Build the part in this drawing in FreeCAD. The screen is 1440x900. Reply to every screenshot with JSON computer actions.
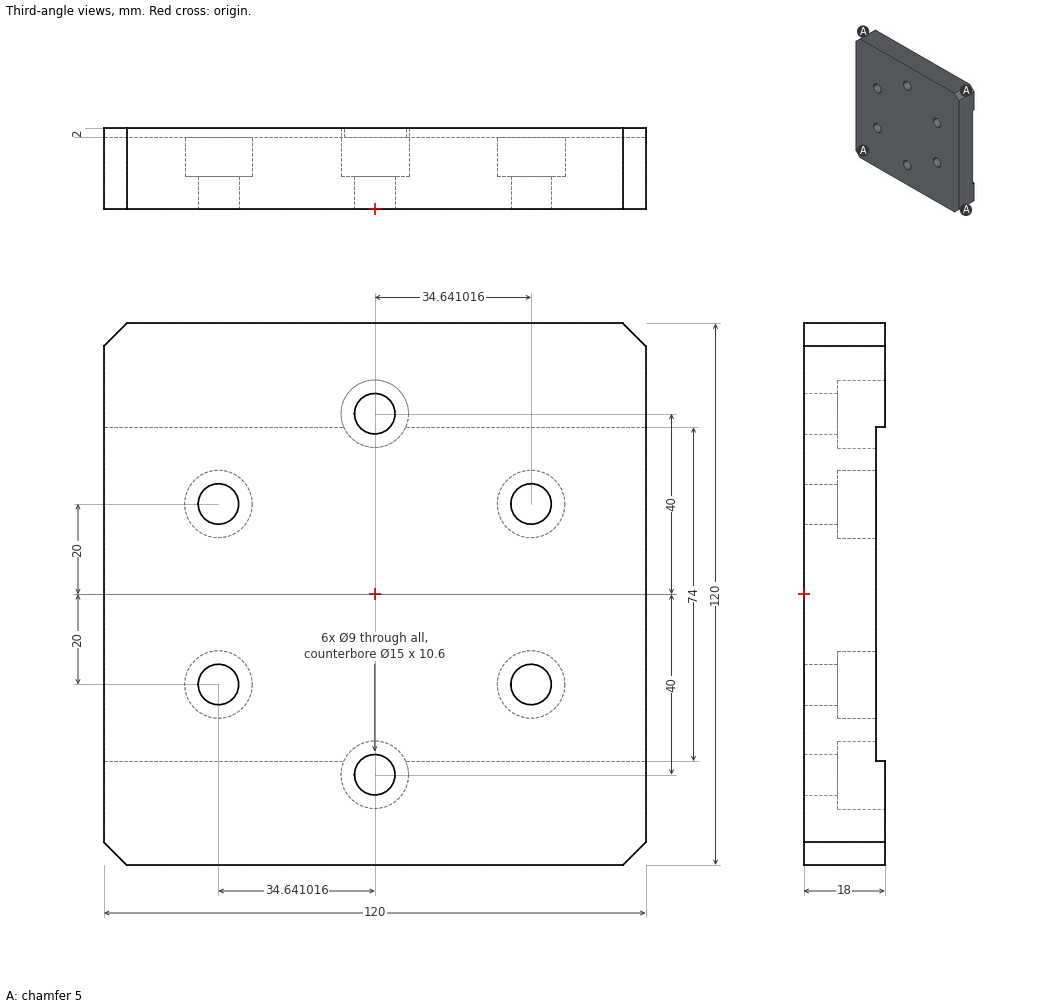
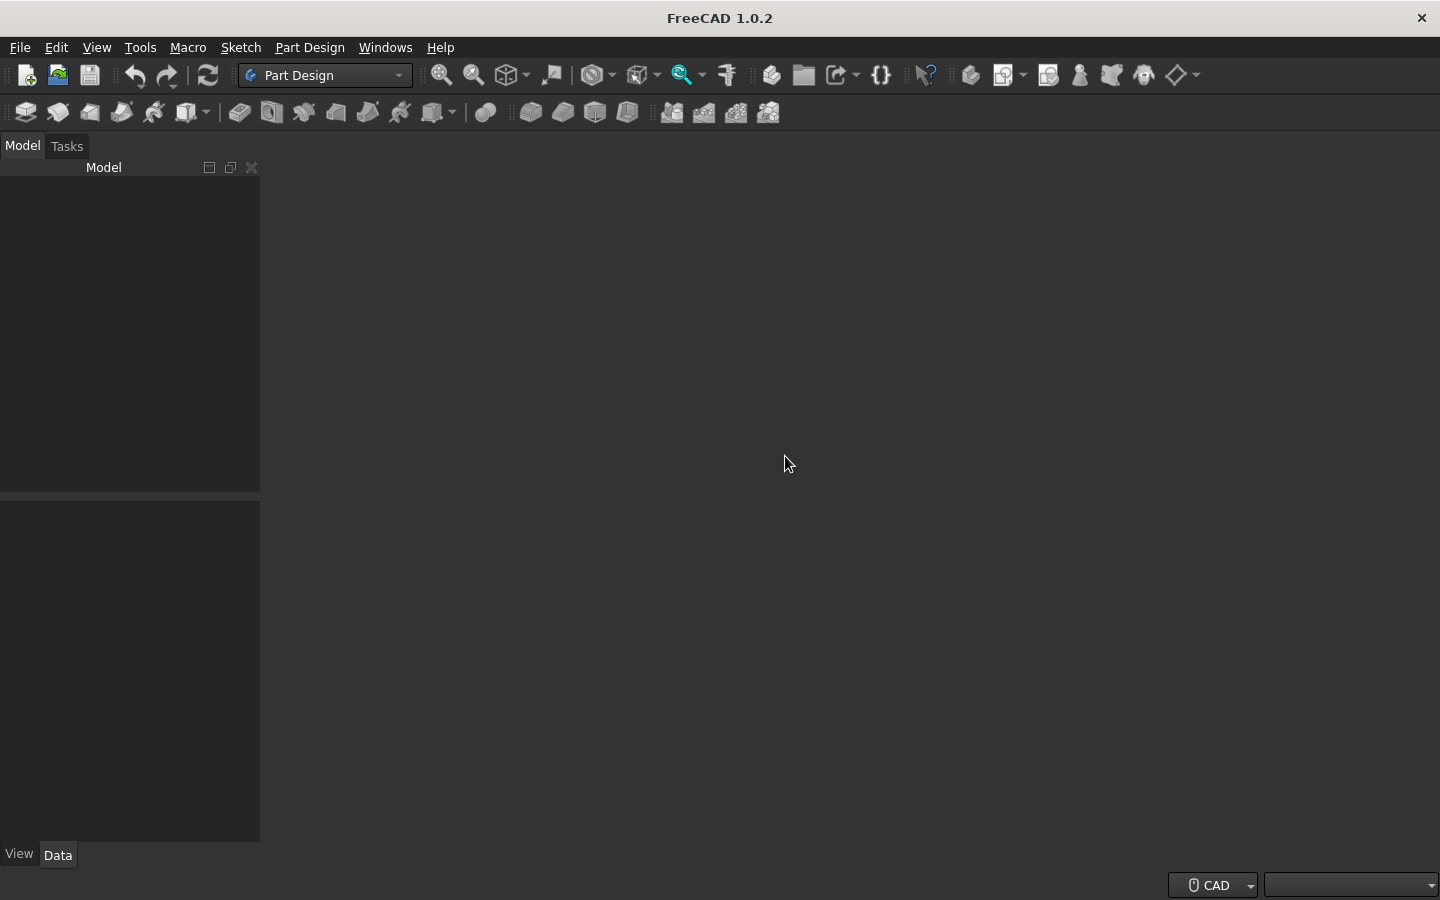
{"action": "left_click", "coordinate": [26, 76]}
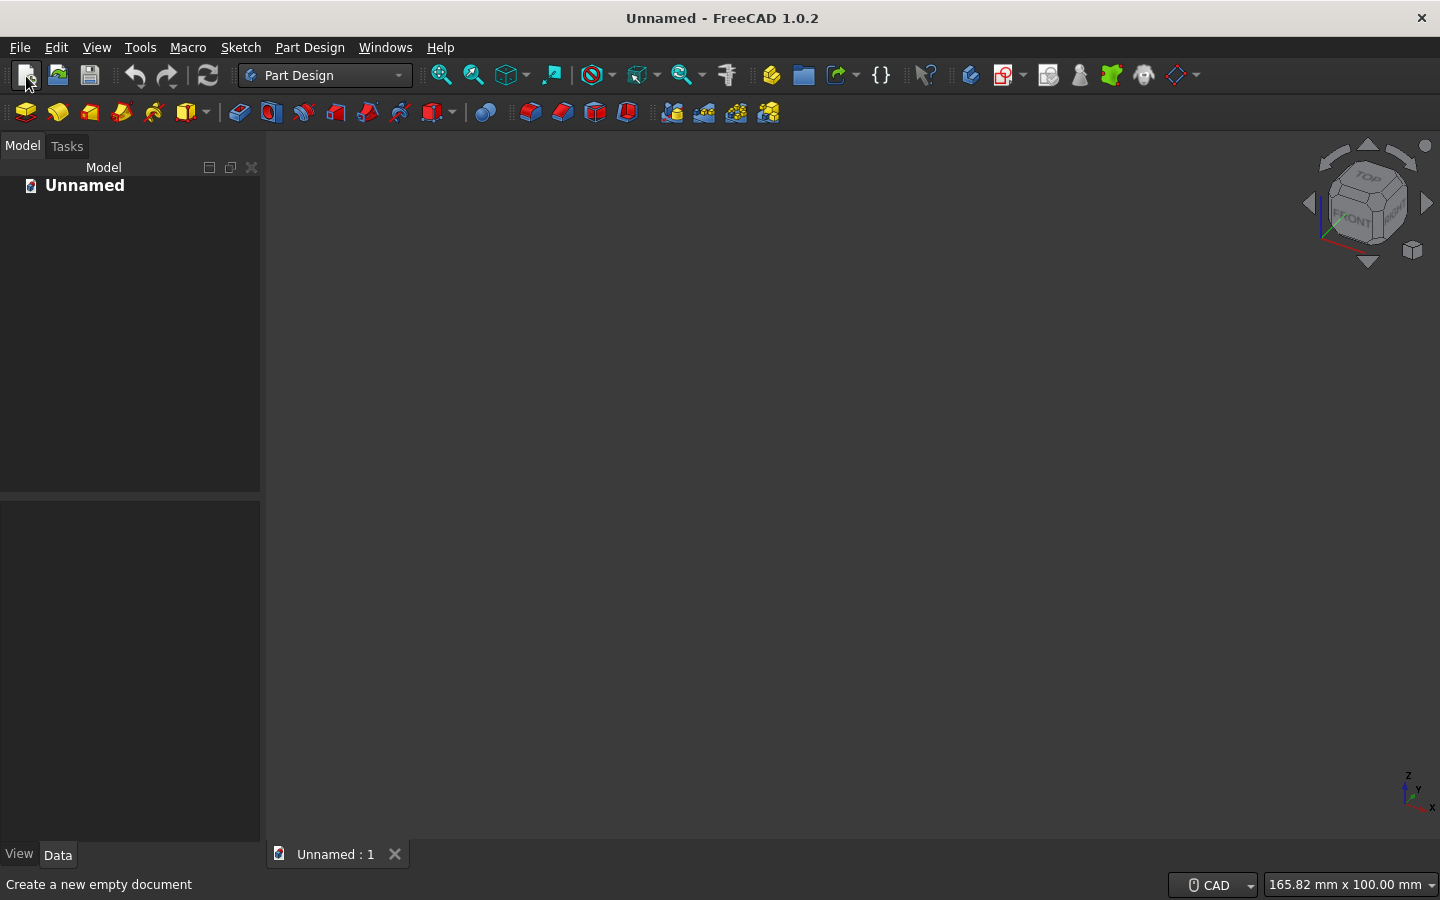
{"action": "left_click", "coordinate": [1004, 76]}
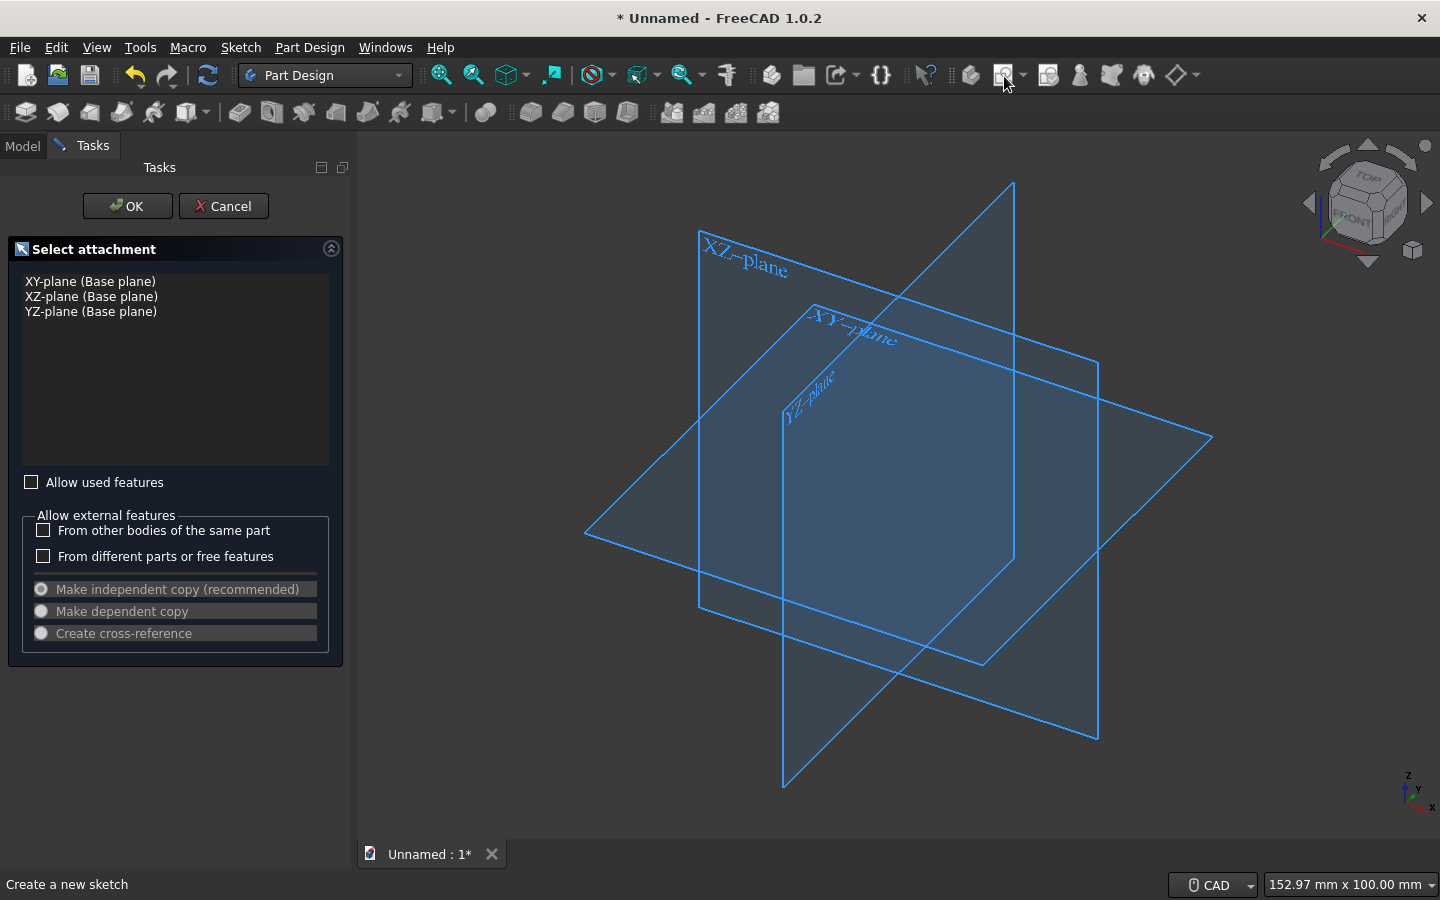
{"action": "left_click", "coordinate": [82, 296]}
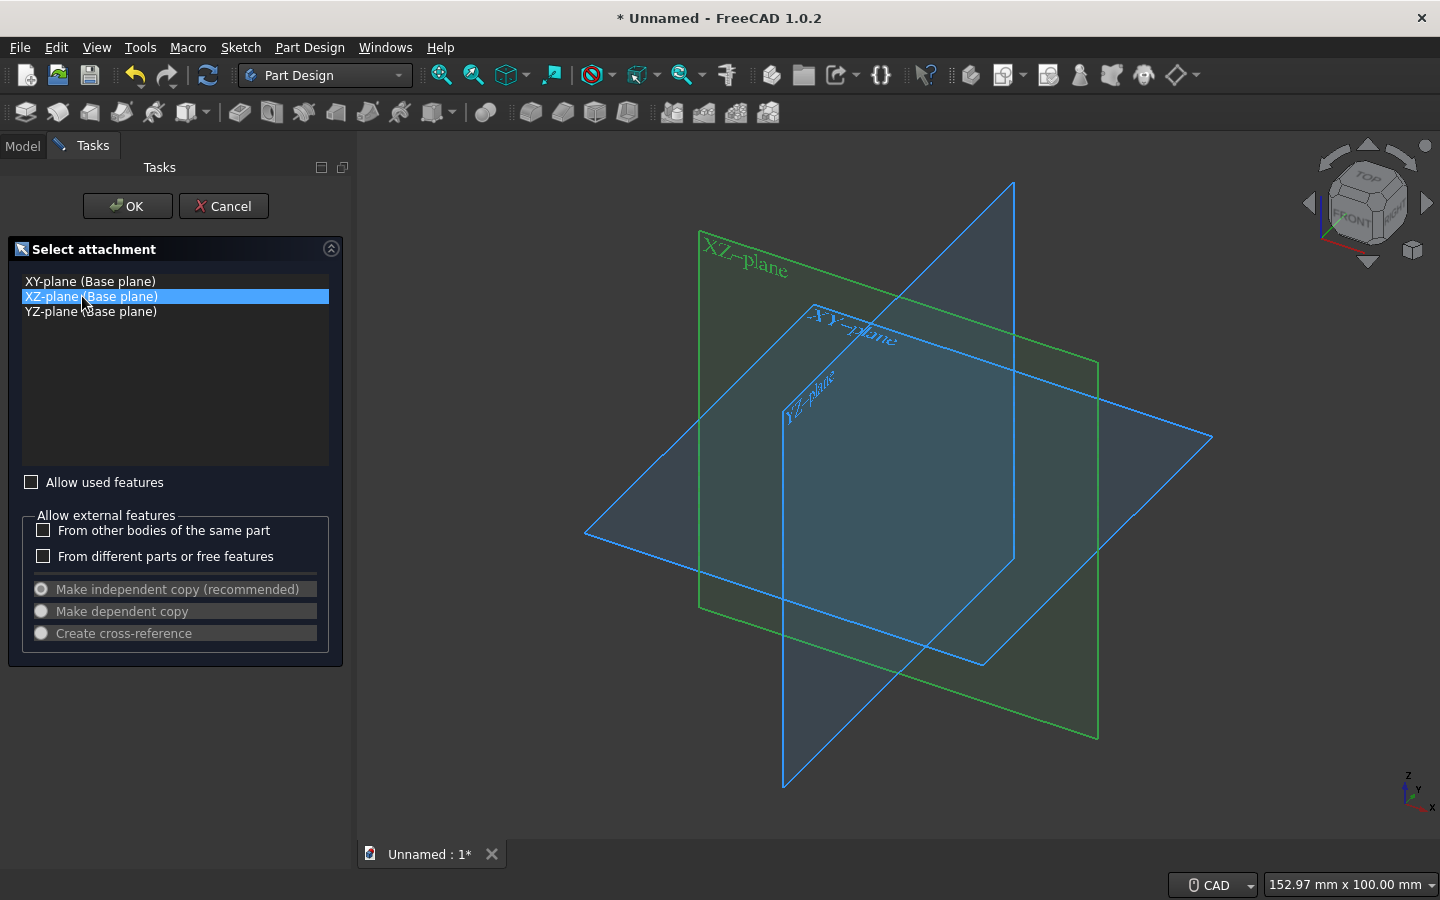
{"action": "left_click", "coordinate": [128, 206]}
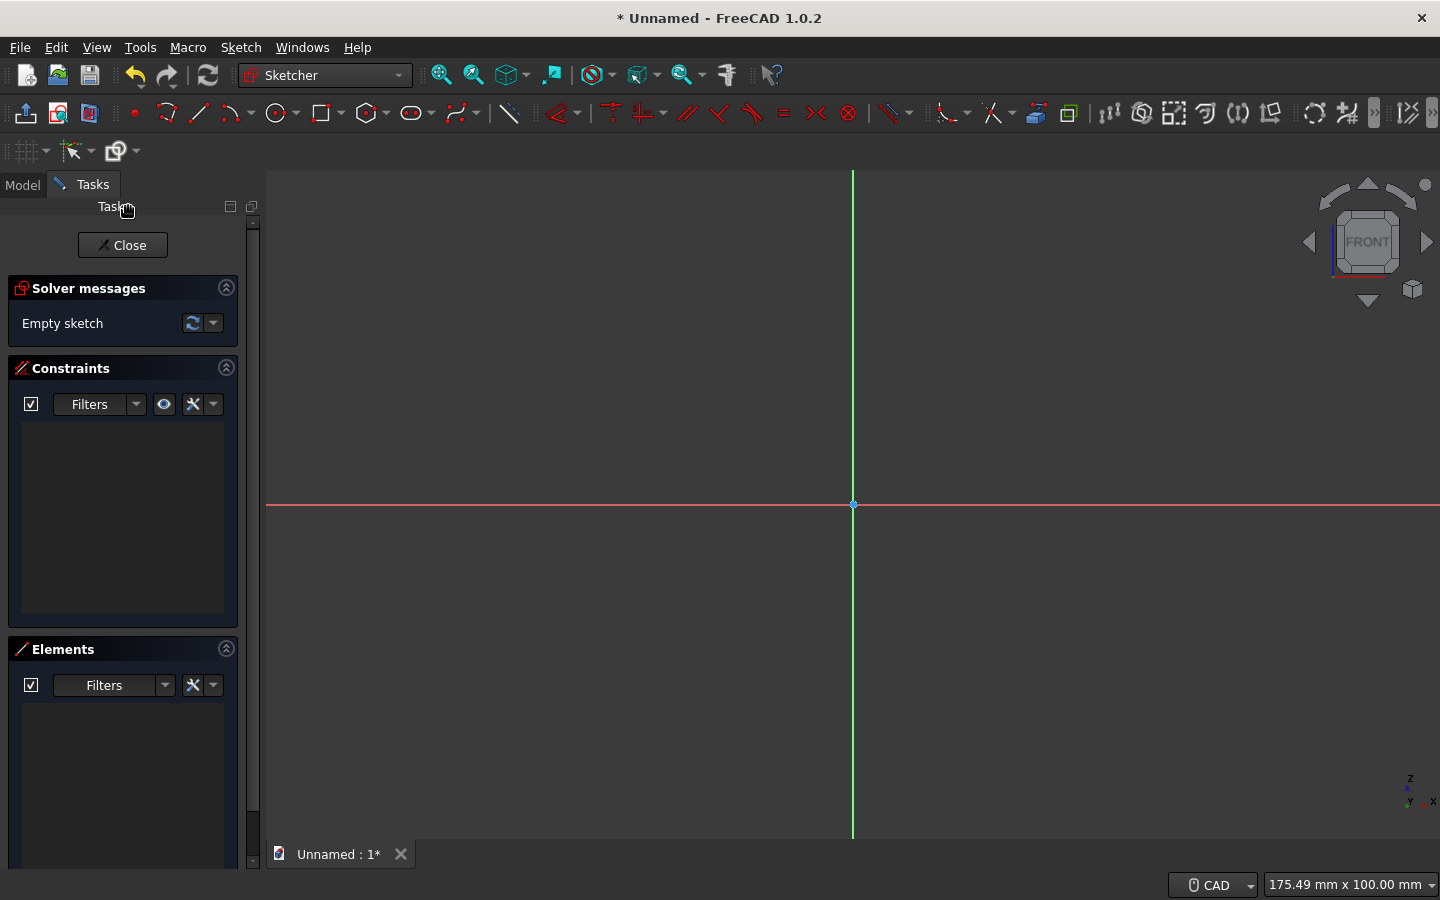
{"action": "scroll", "coordinate": [701, 504], "scroll_direction": "down", "scroll_amount": 3}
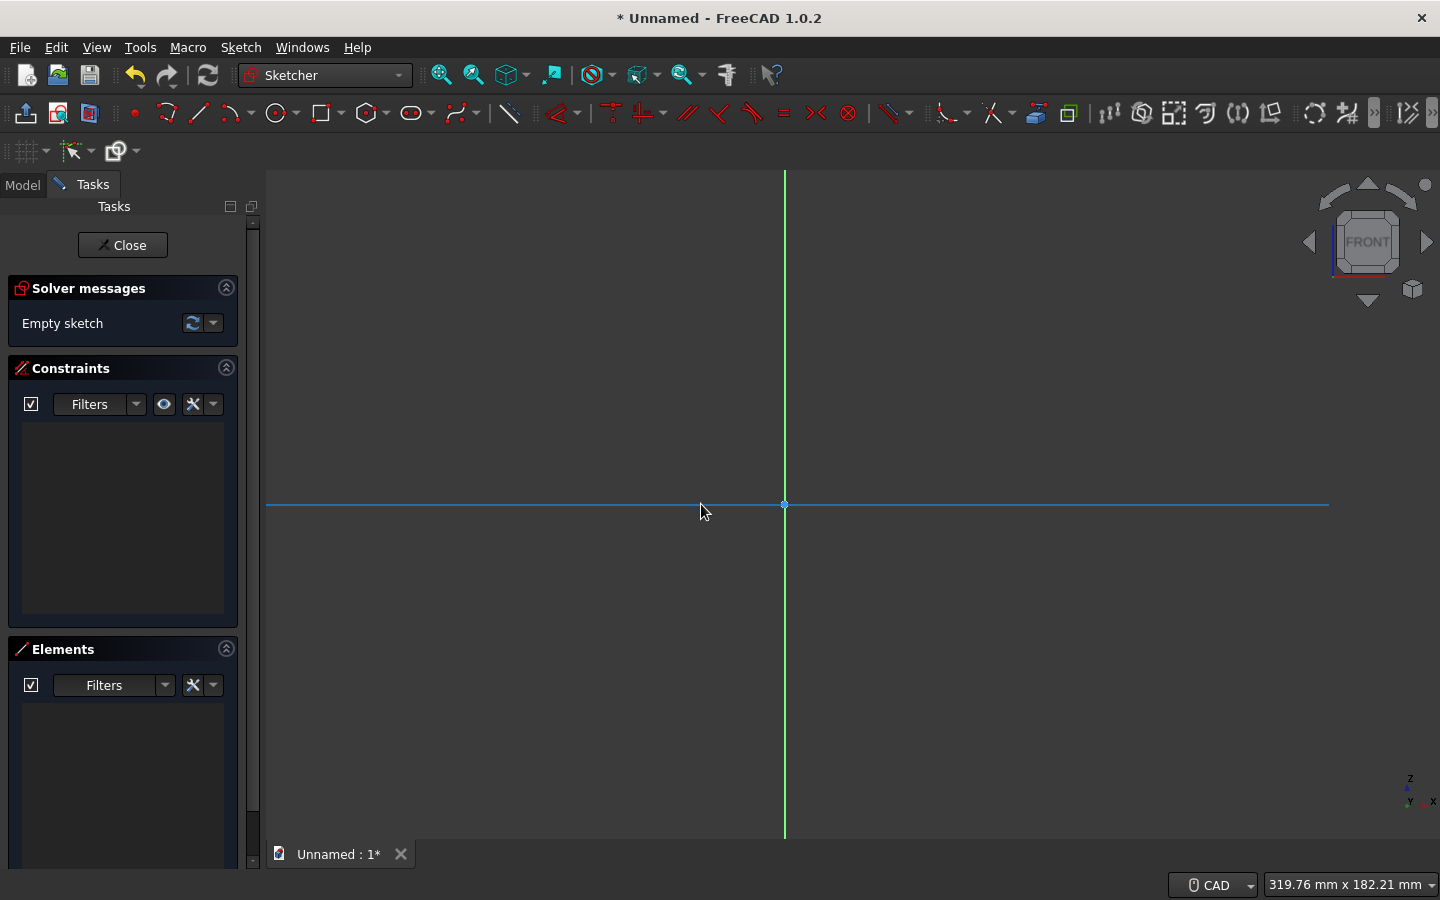
{"action": "key", "text": "g v"}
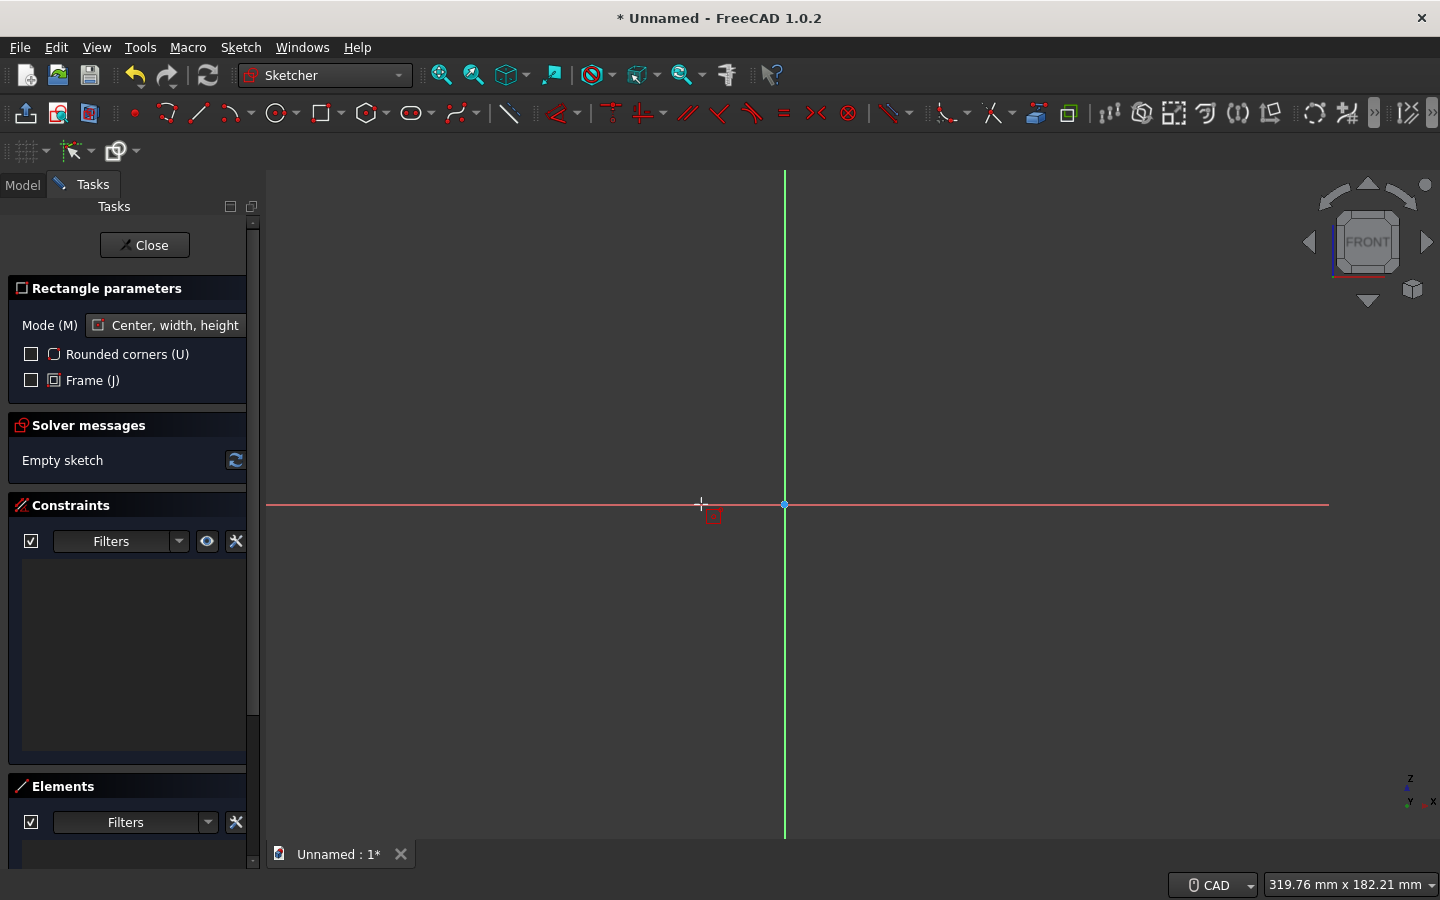
{"action": "left_click", "coordinate": [785, 504]}
{"action": "mouse_move", "coordinate": [1005, 284]}